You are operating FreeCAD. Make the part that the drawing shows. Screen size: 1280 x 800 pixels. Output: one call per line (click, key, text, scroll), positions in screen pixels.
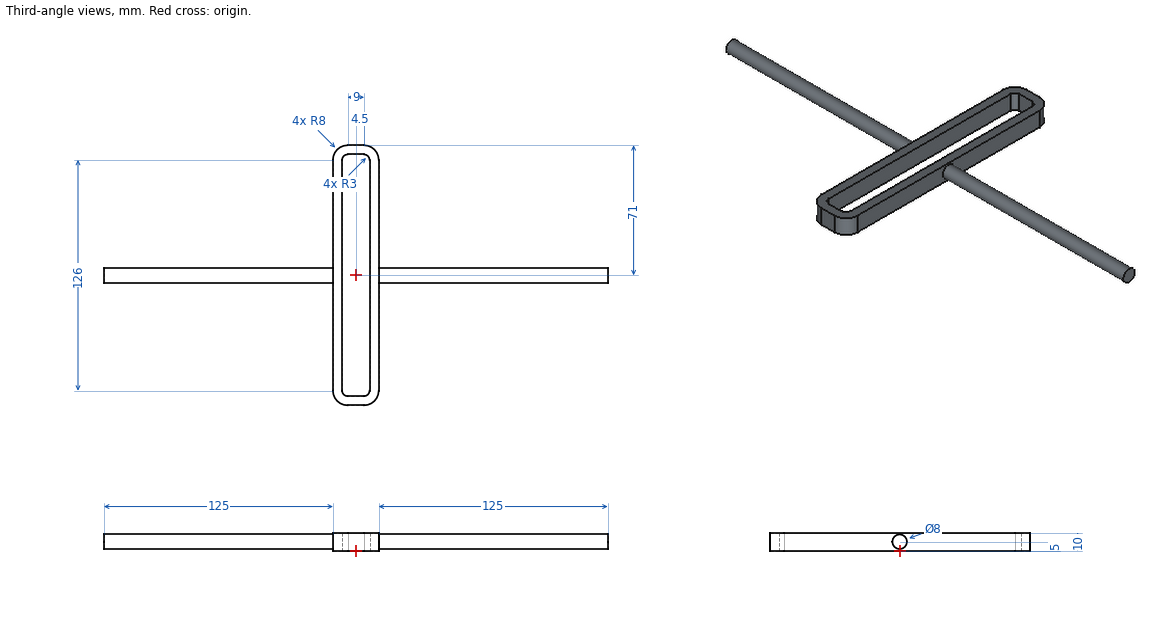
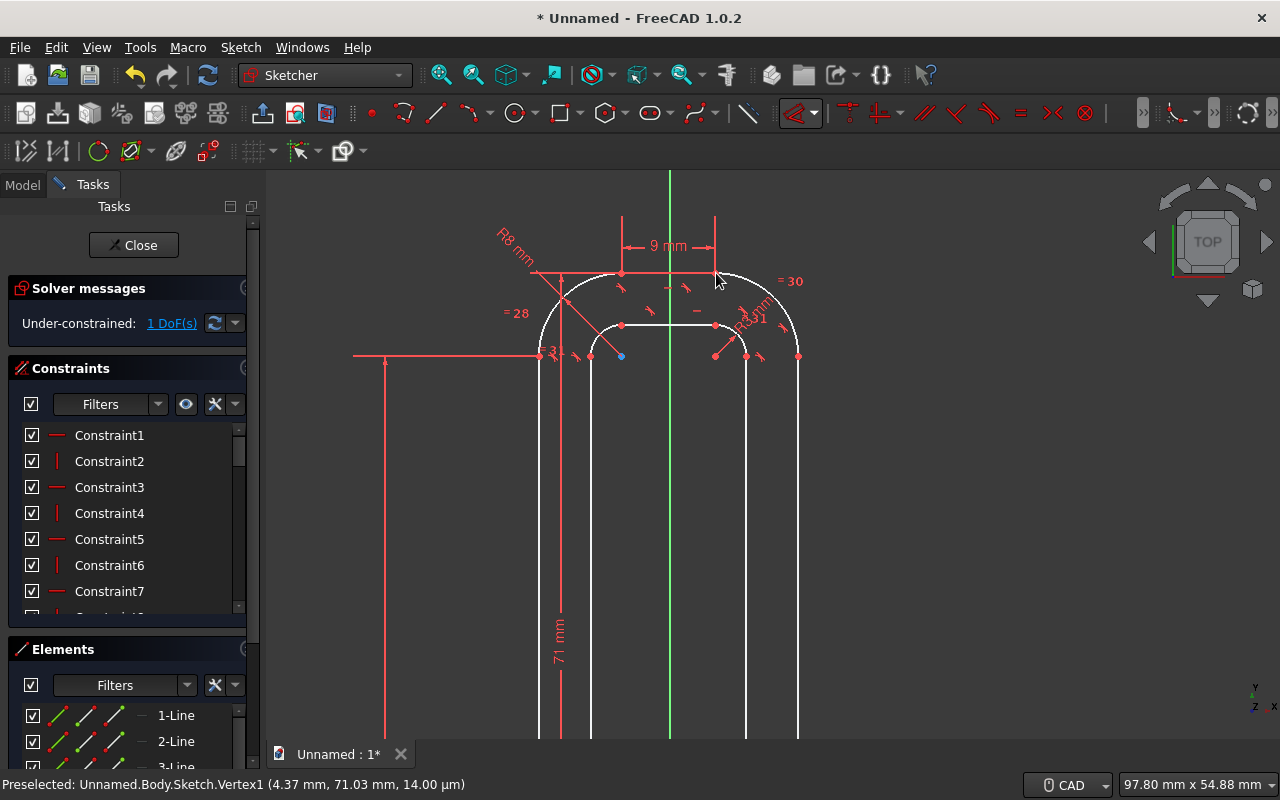
click(715, 273)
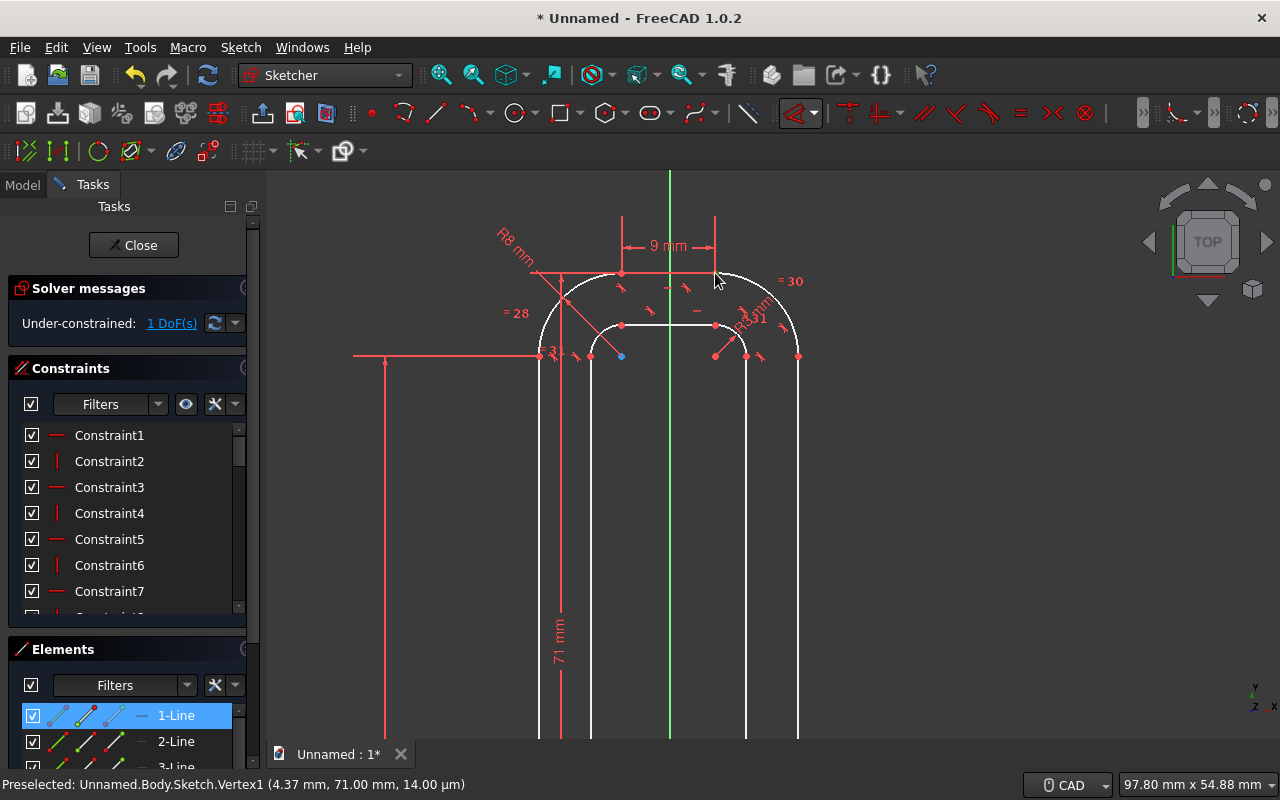
click(816, 114)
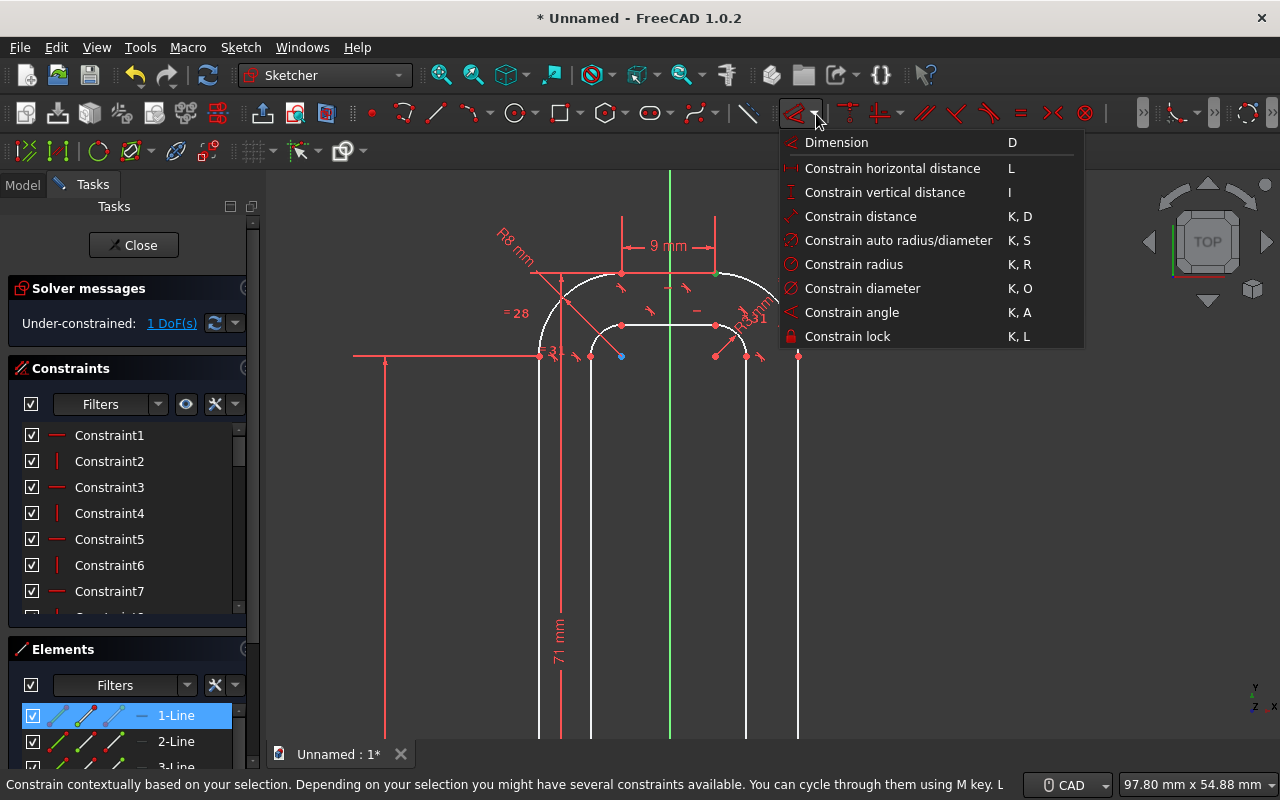
click(932, 168)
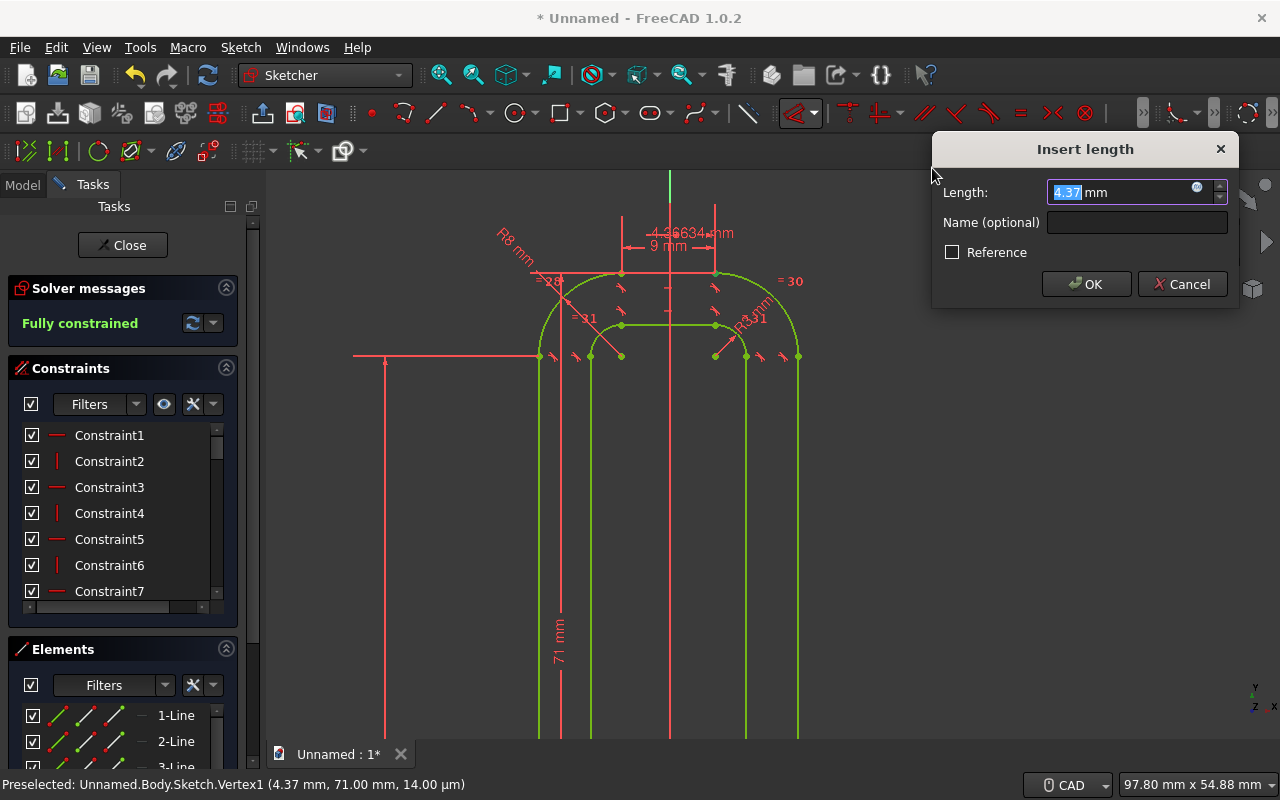
text(4.5)
key(Return)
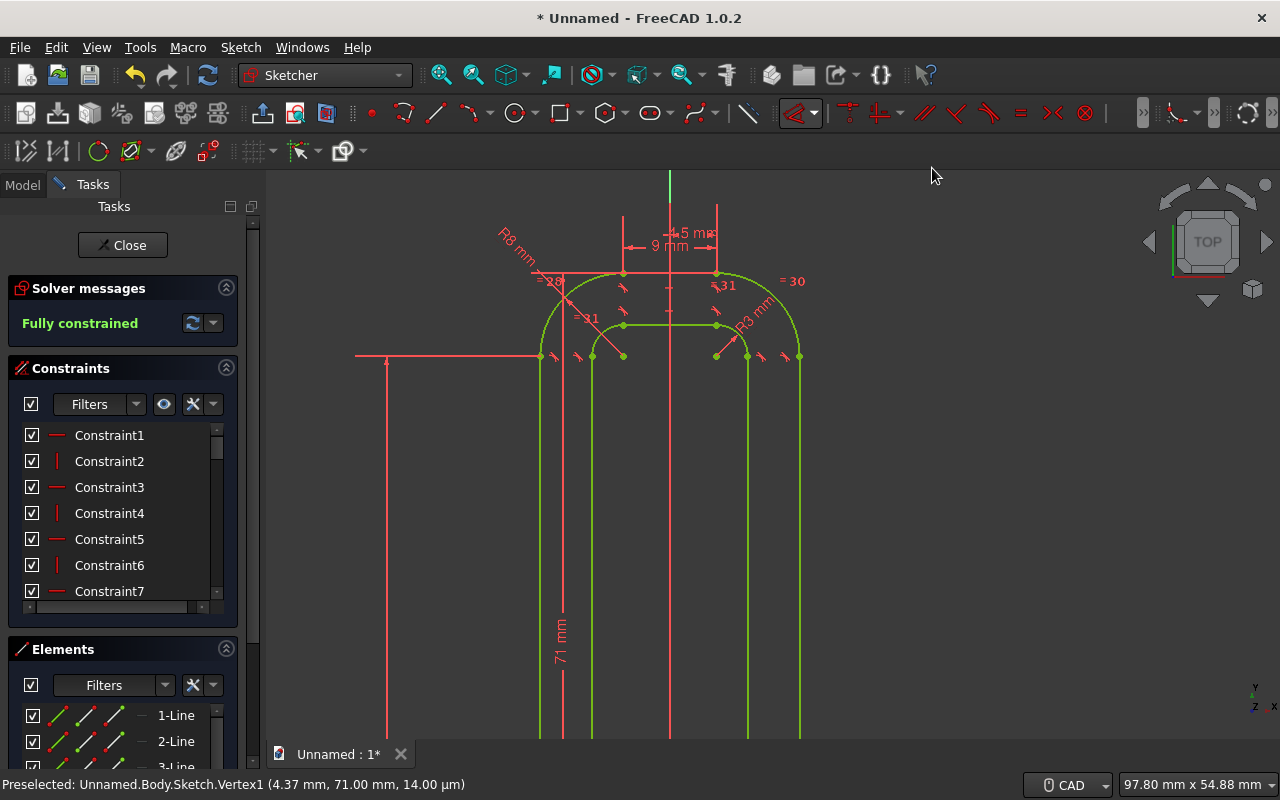
click(123, 245)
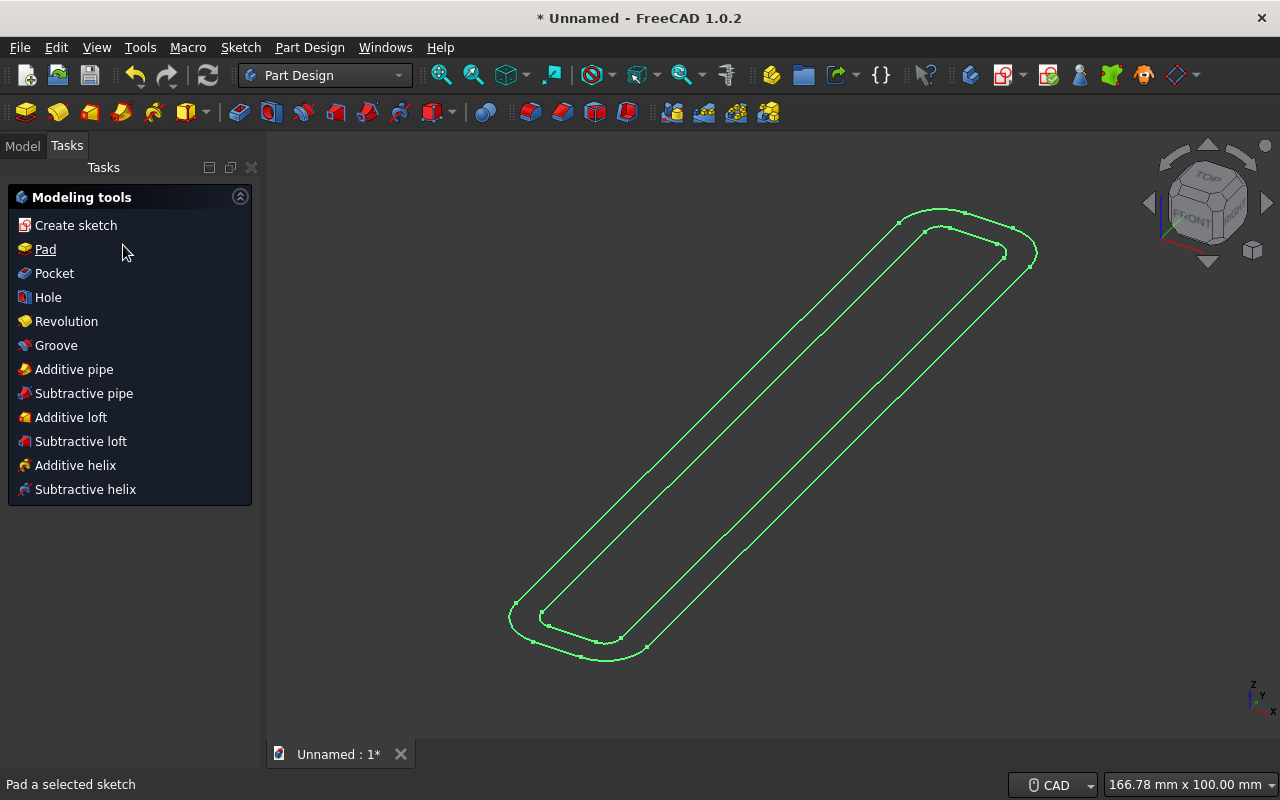
click(26, 112)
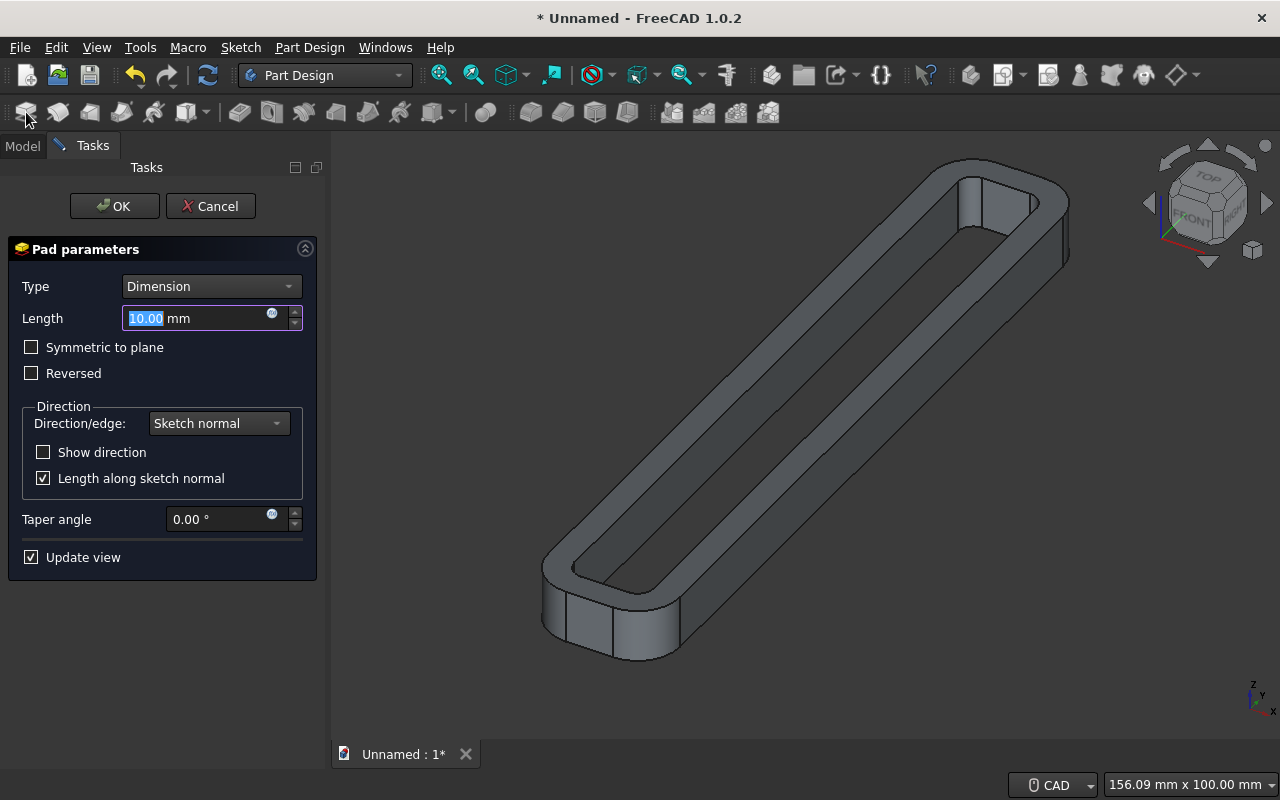
text(10)
key(Tab)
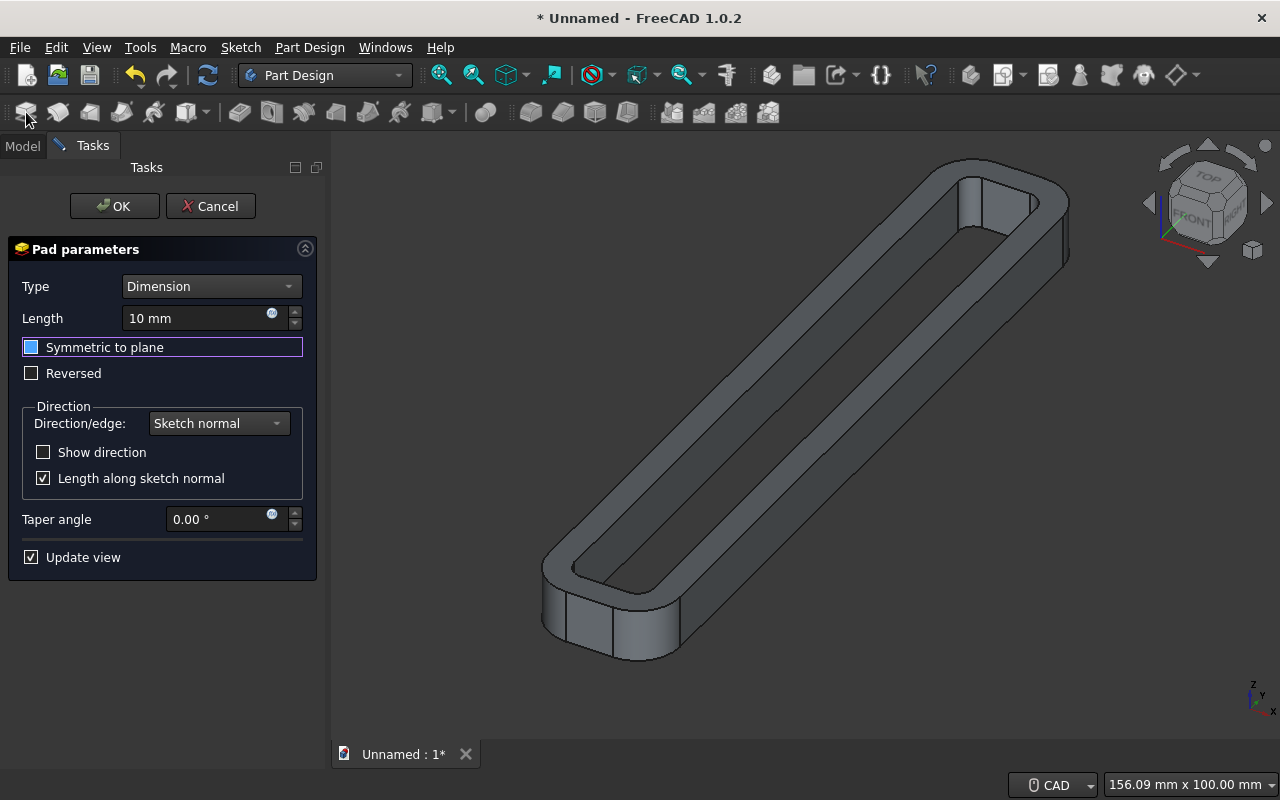
click(115, 206)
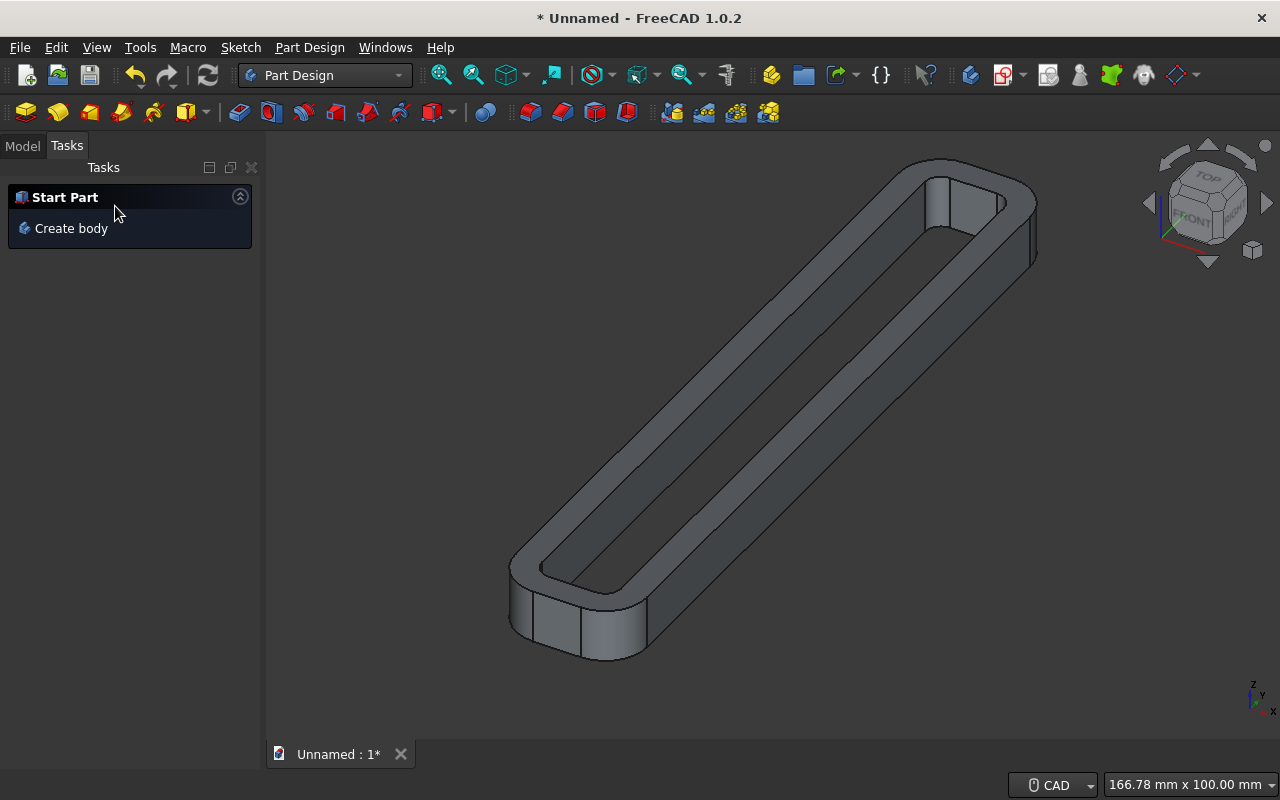
click(1003, 268)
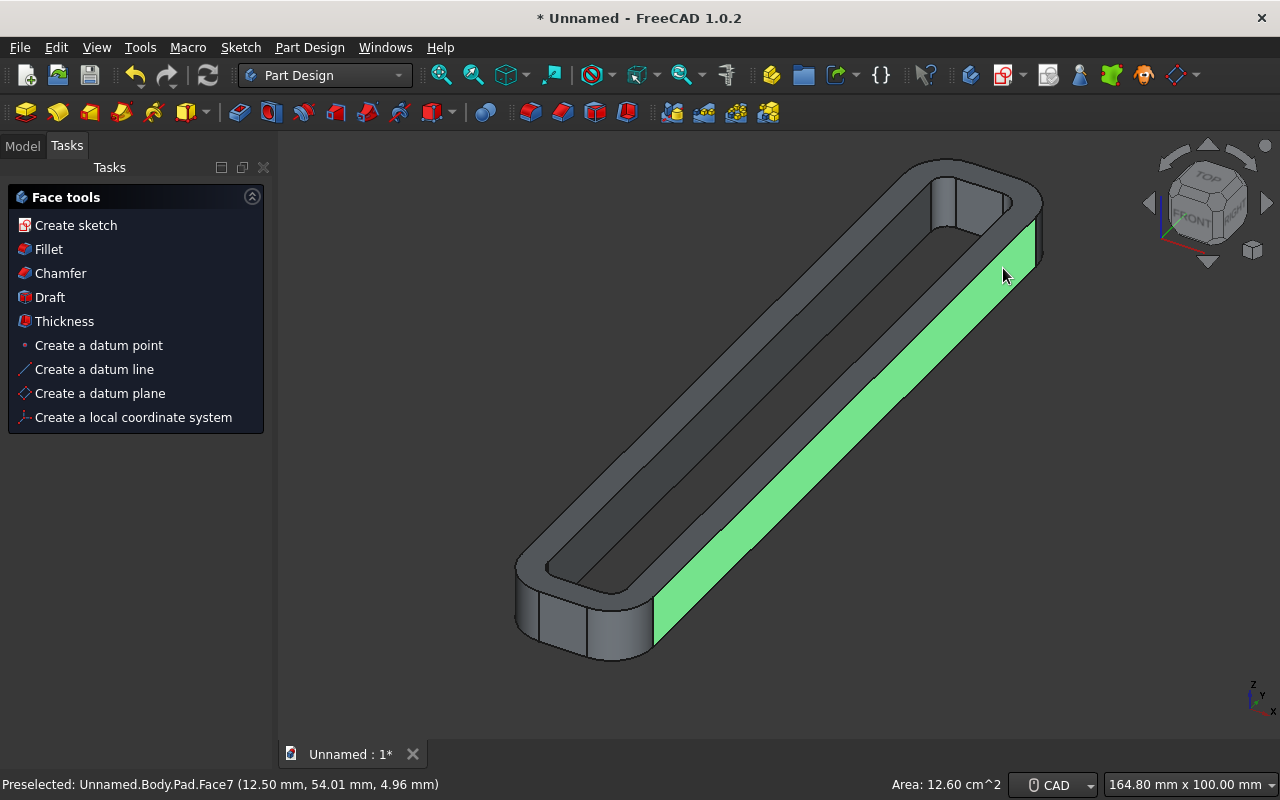
click(1004, 76)